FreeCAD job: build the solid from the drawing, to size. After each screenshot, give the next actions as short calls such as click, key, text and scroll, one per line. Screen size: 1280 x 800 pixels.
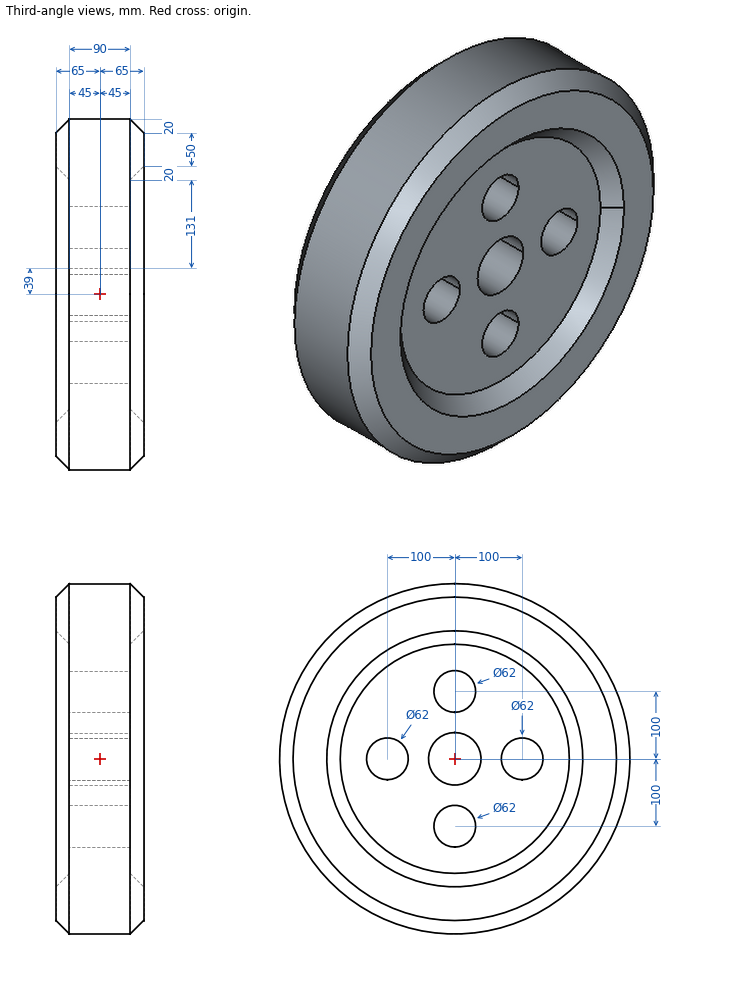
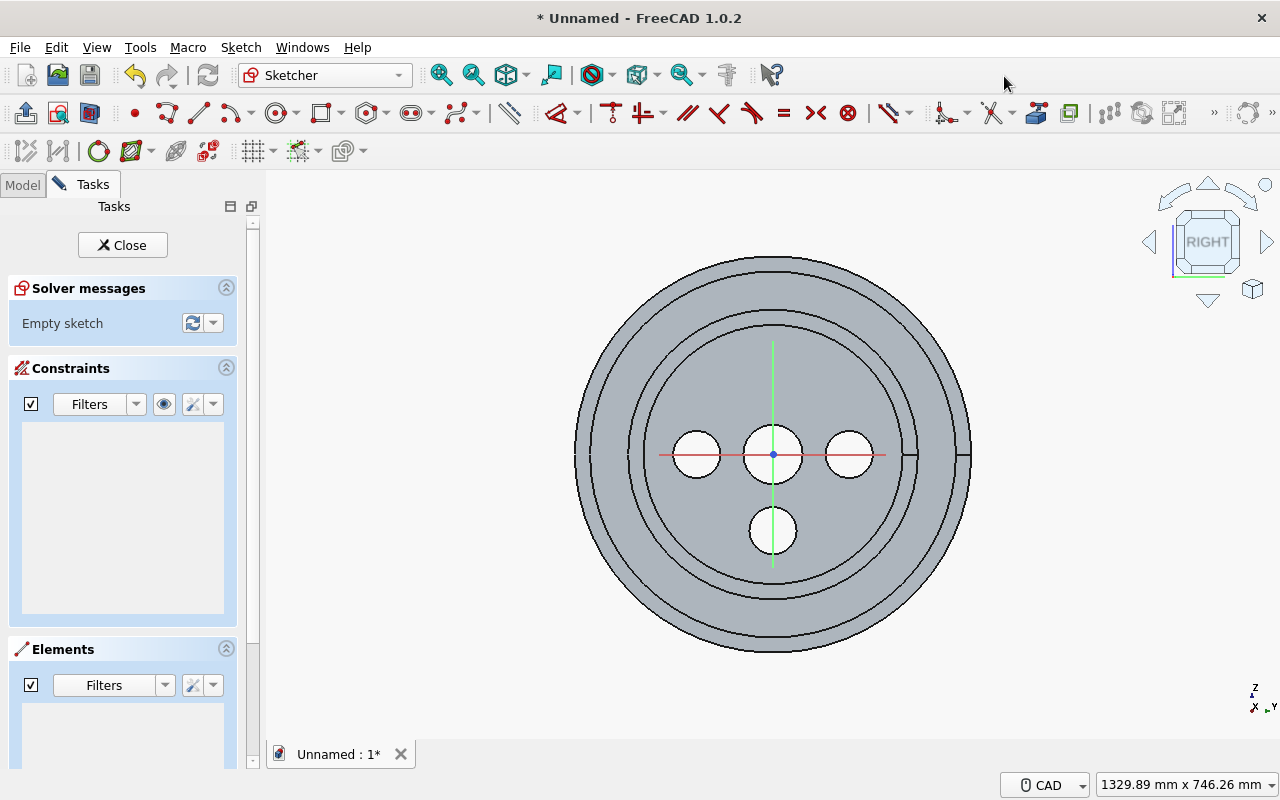
scroll(803, 383, up, 6)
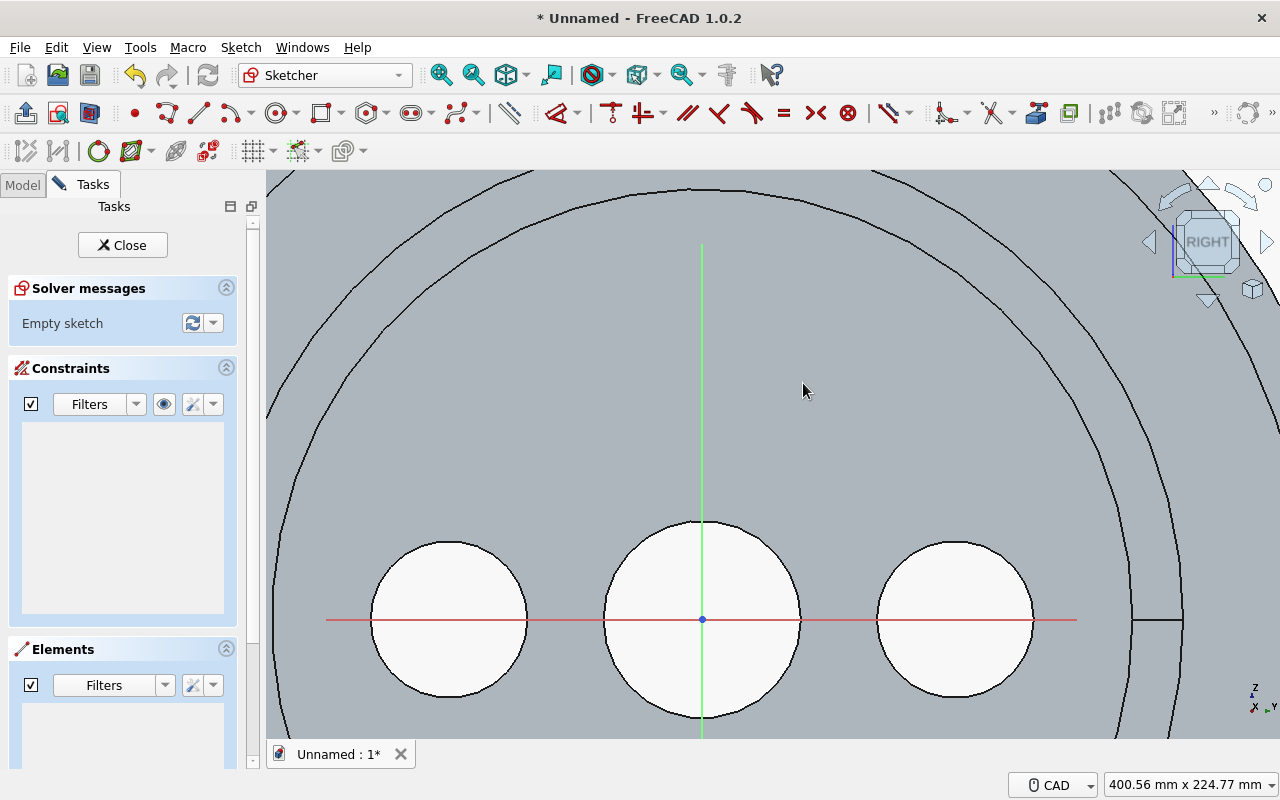
click(276, 114)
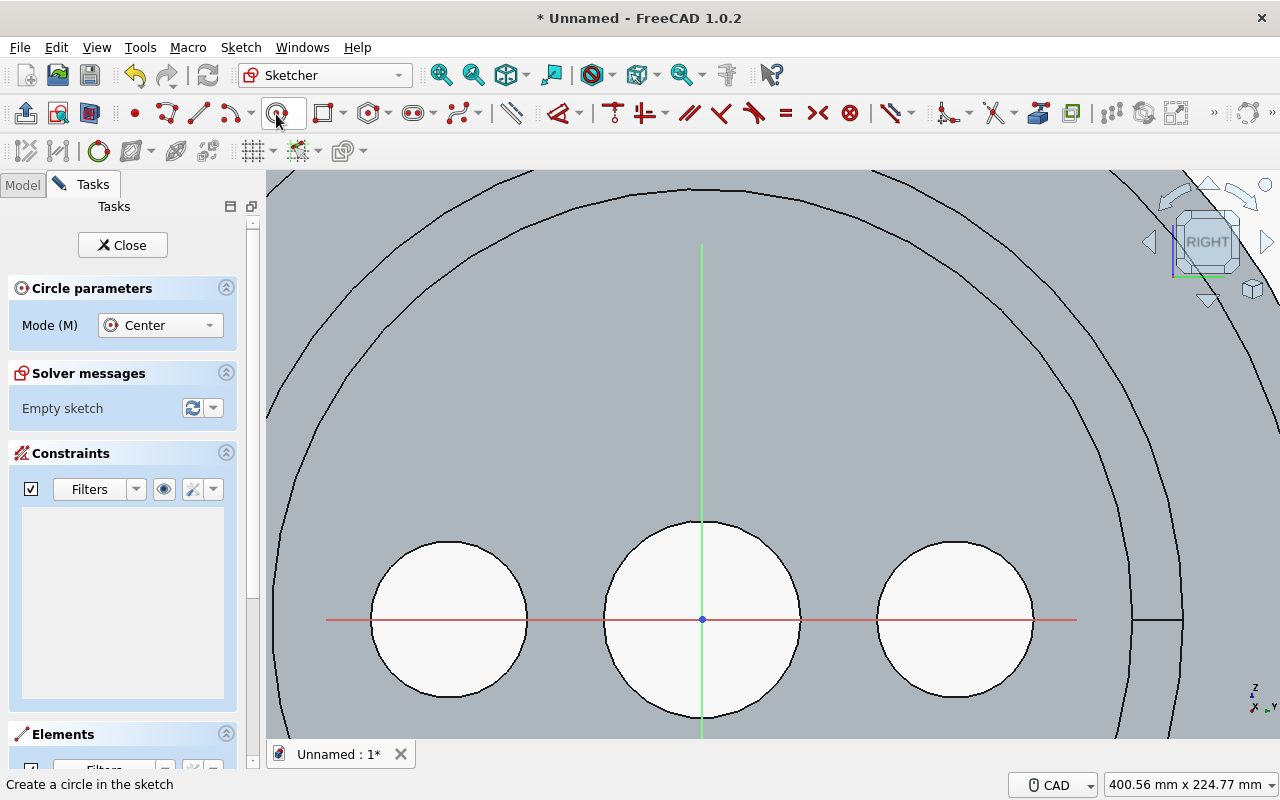
click(702, 366)
click(758, 311)
key(Escape)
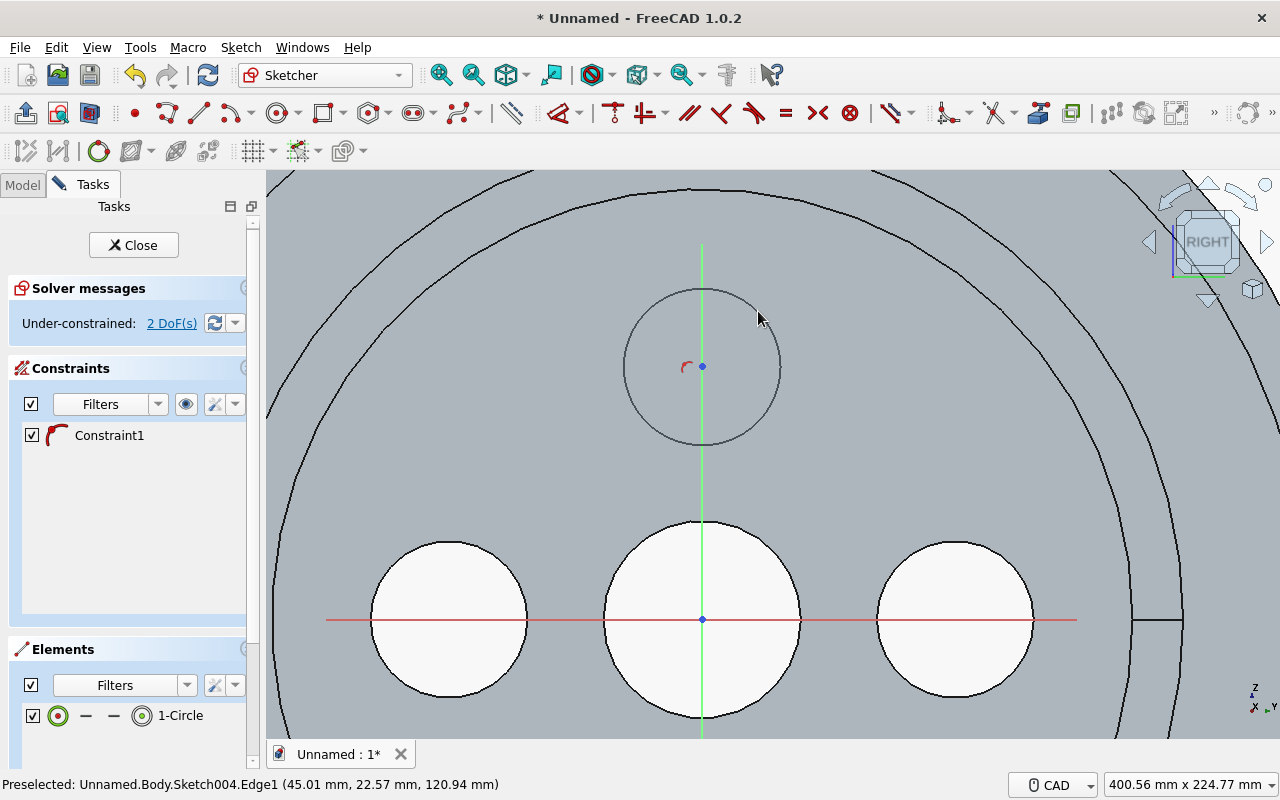
key(d)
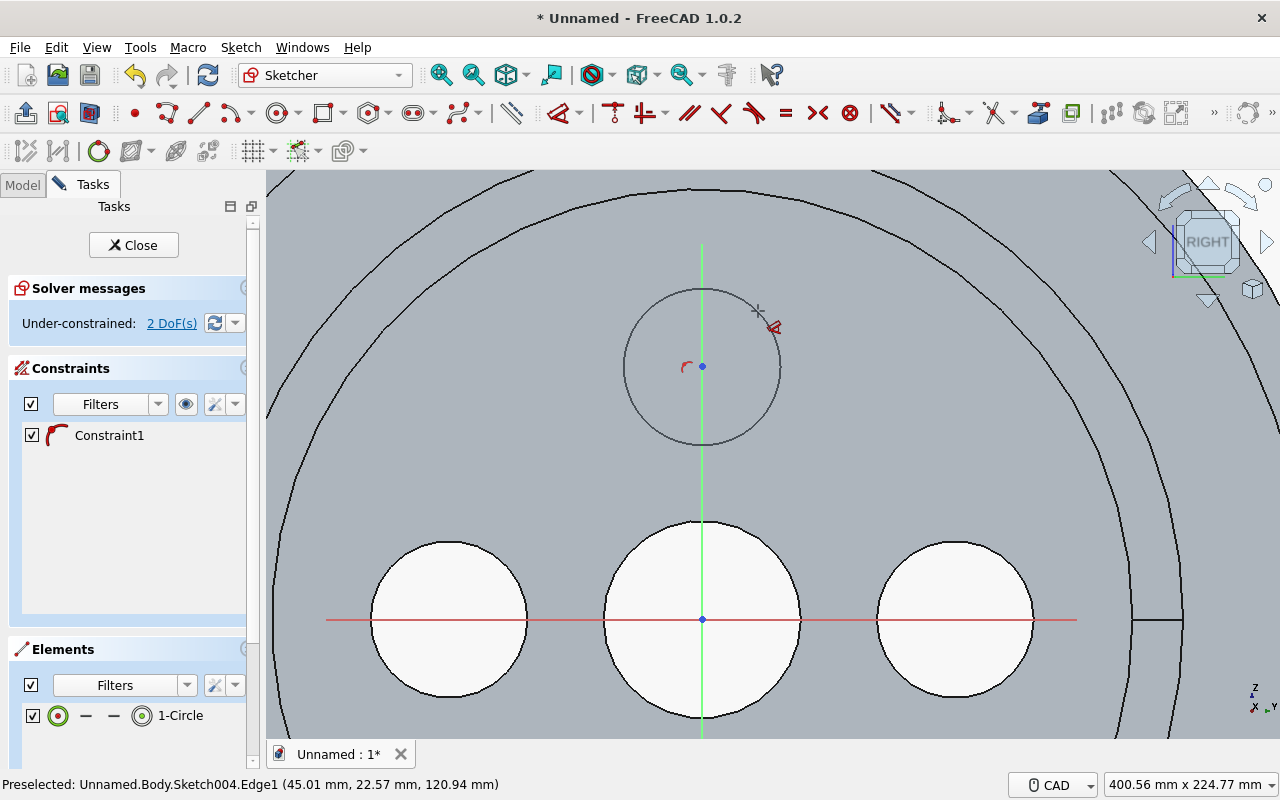
click(757, 311)
click(779, 288)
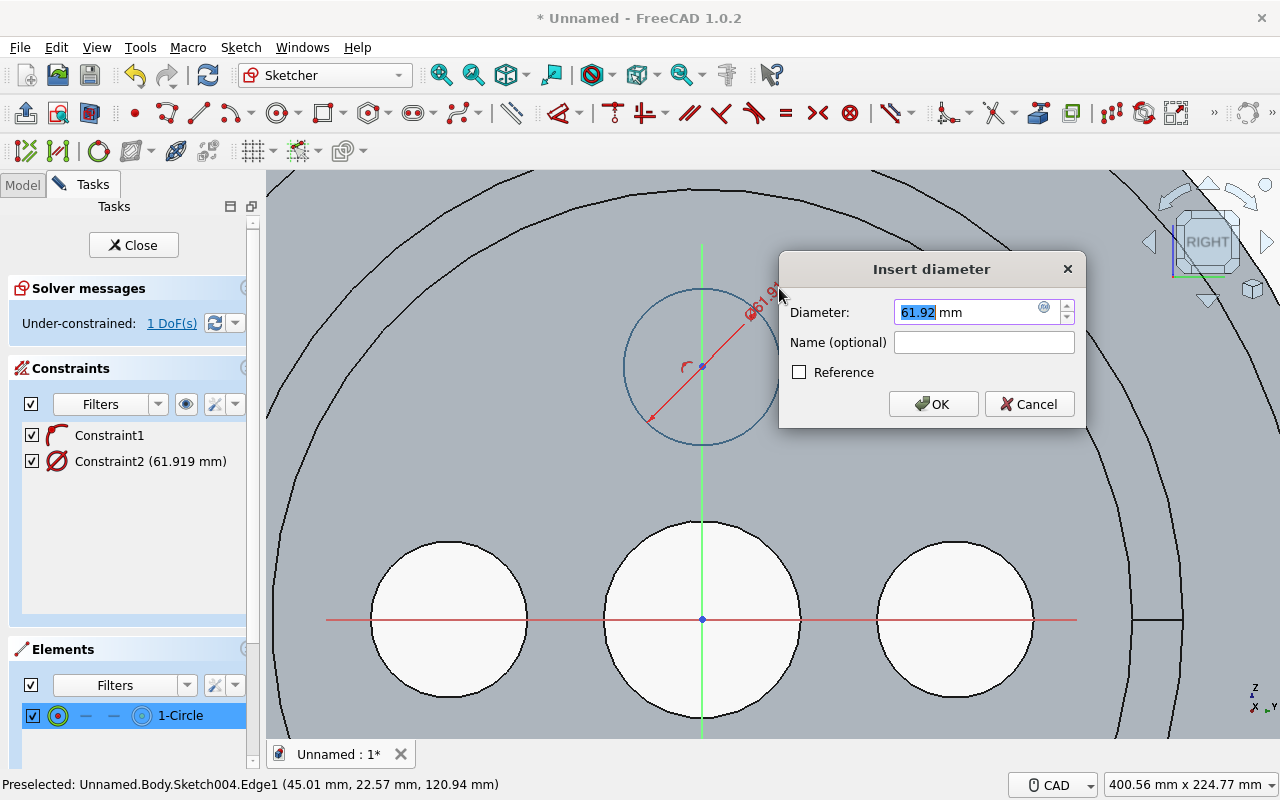
text(62)
key(Return)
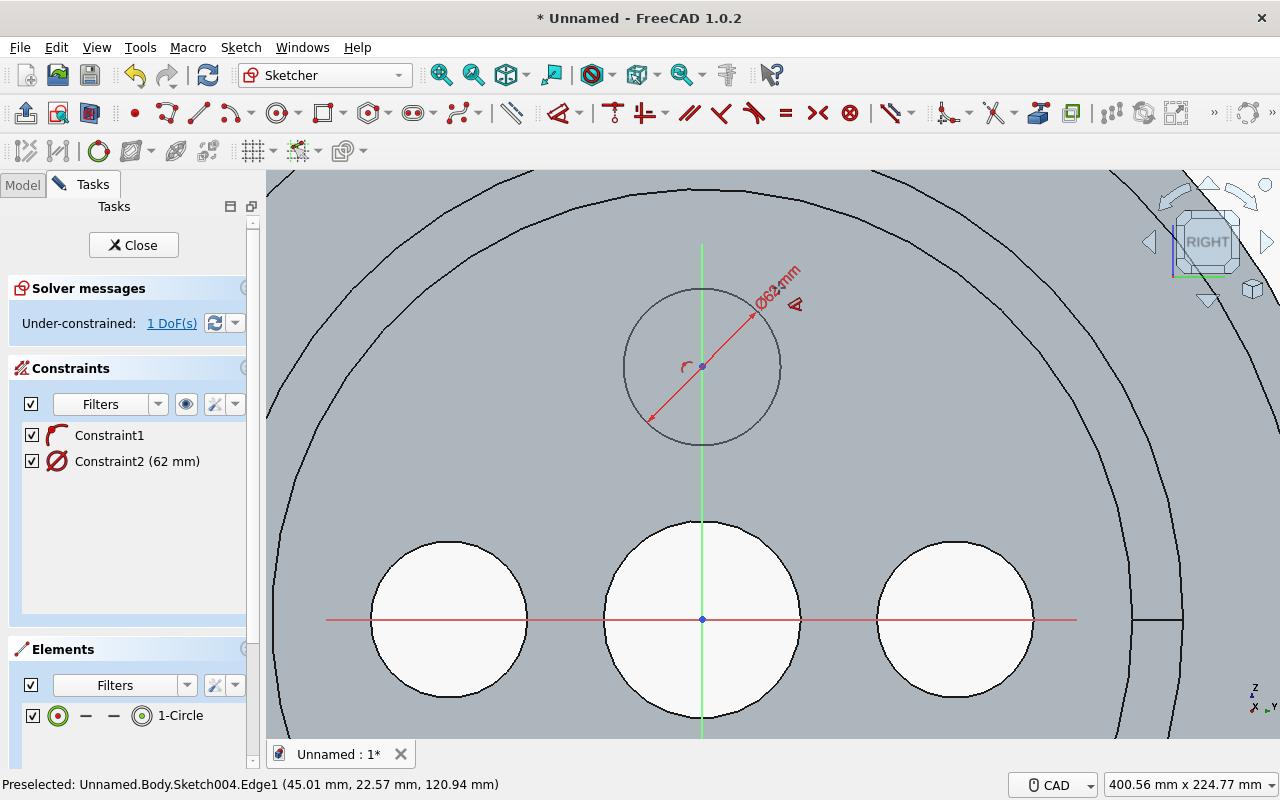
click(702, 367)
click(736, 493)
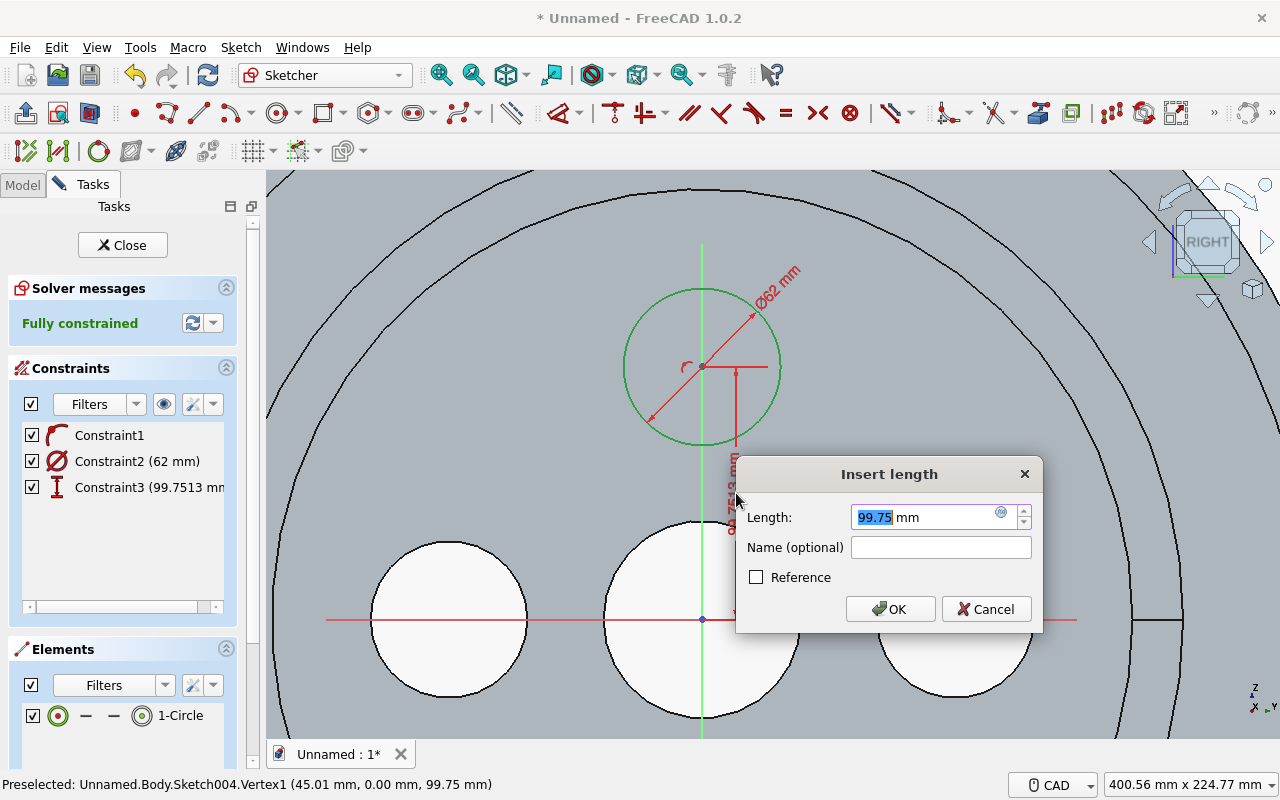
text(100)
key(Return)
key(Escape)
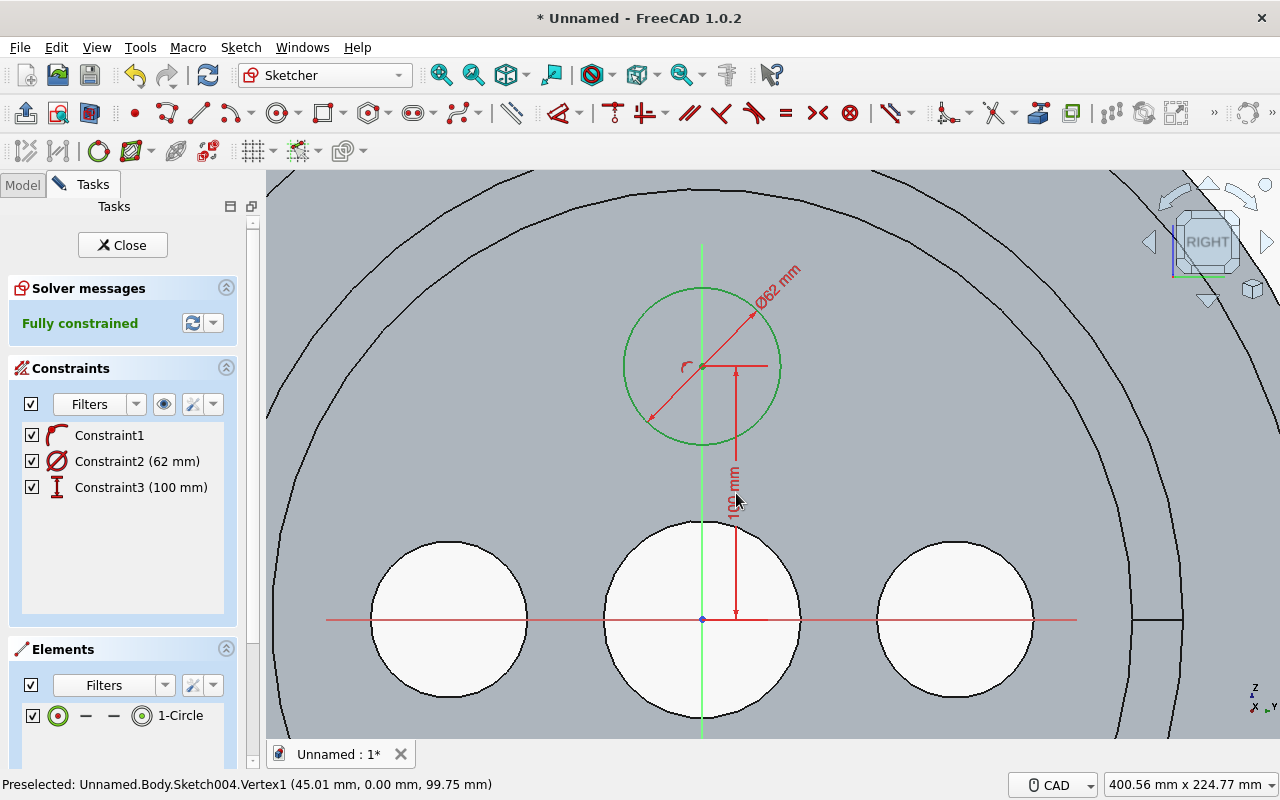
click(123, 245)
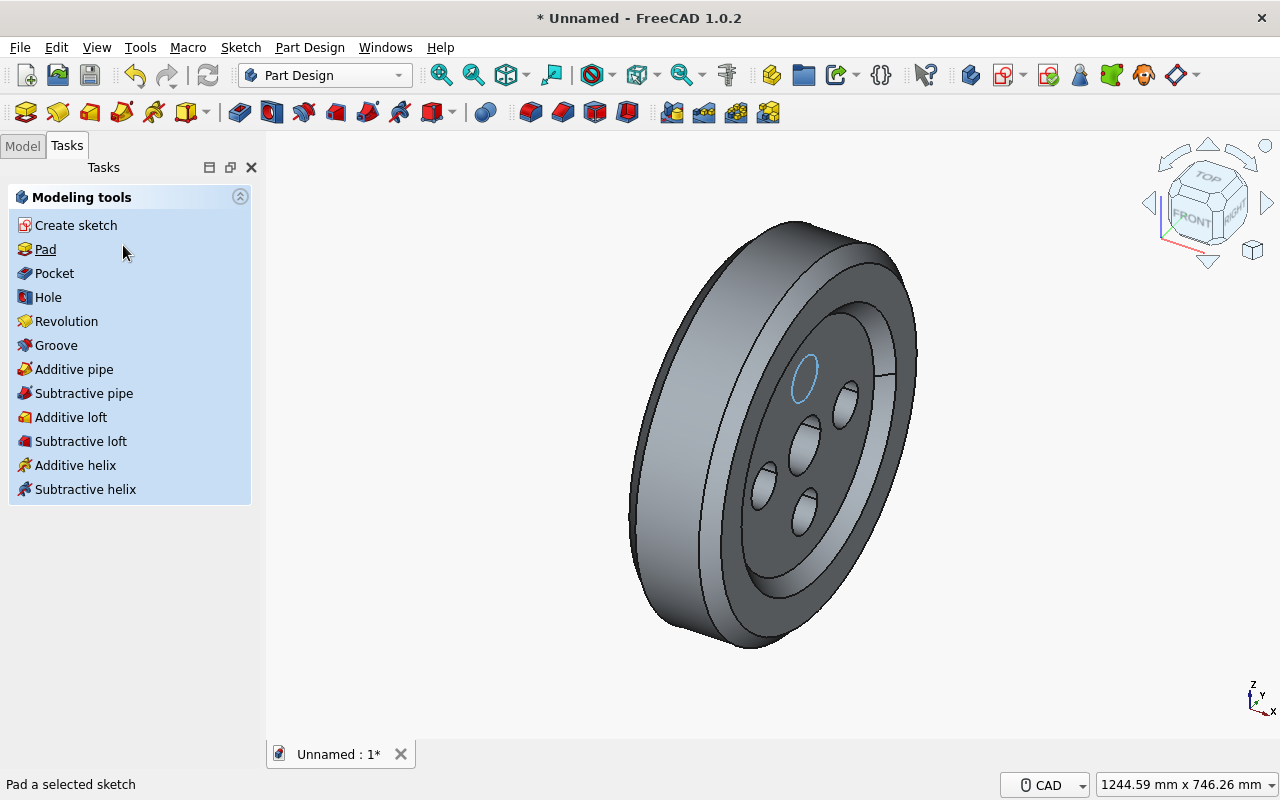
click(240, 112)